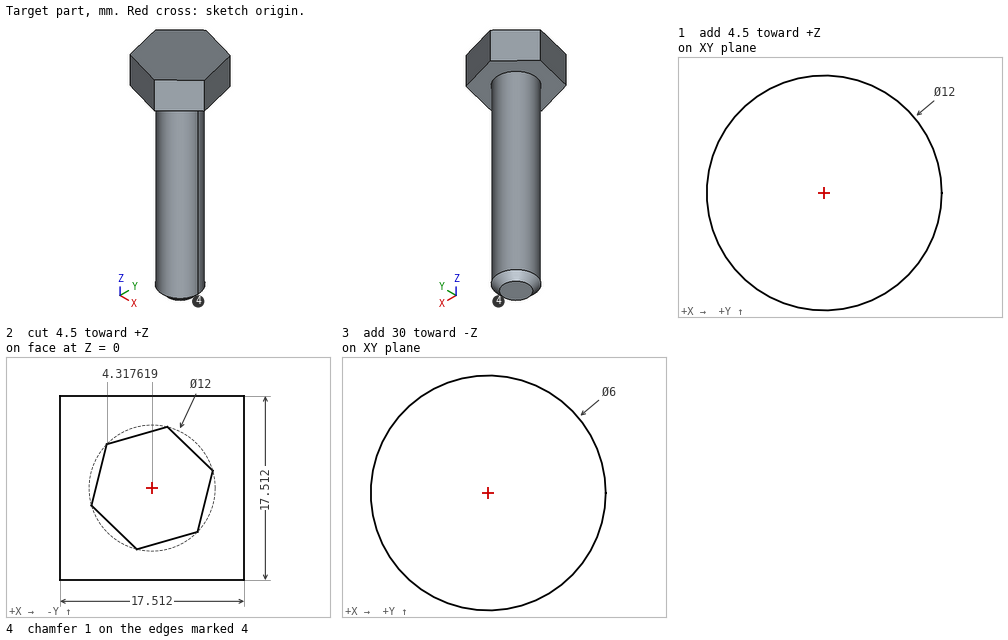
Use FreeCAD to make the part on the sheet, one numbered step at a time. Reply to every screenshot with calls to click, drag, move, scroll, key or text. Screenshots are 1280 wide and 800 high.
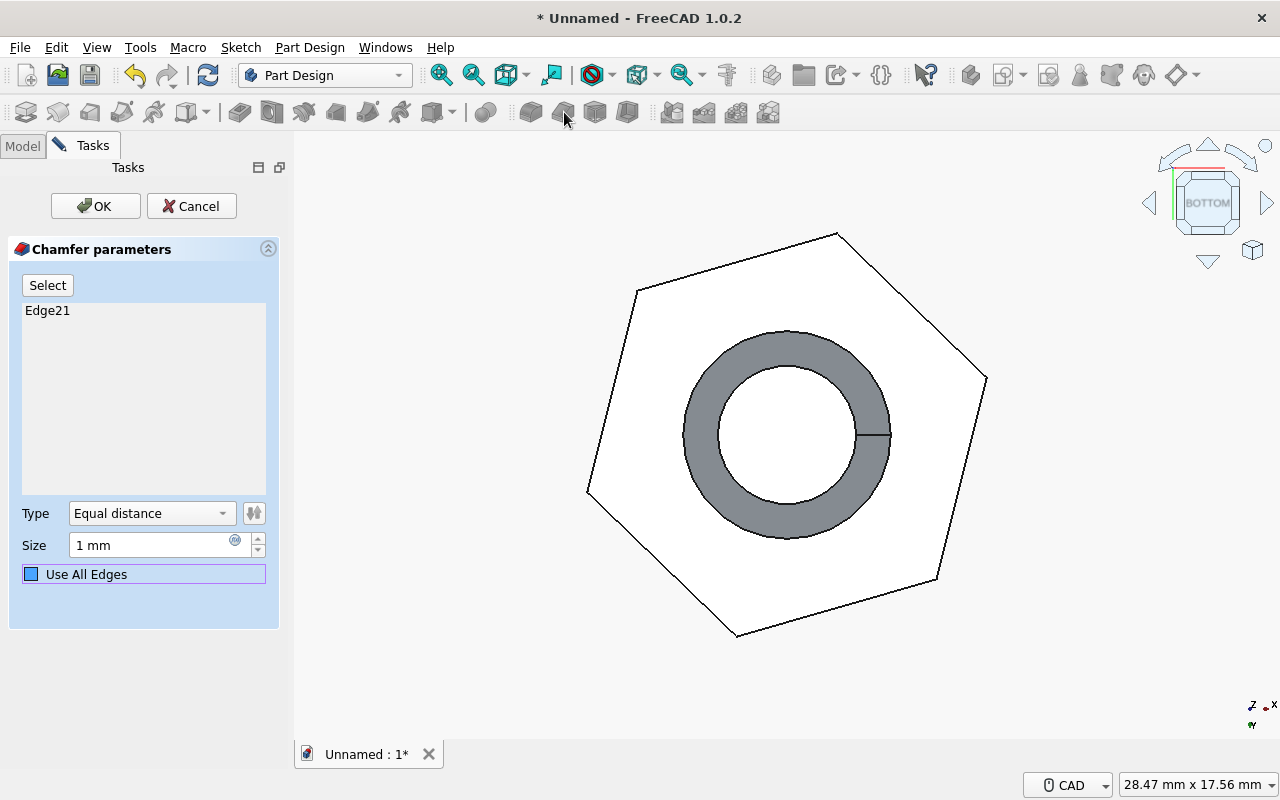
click(96, 206)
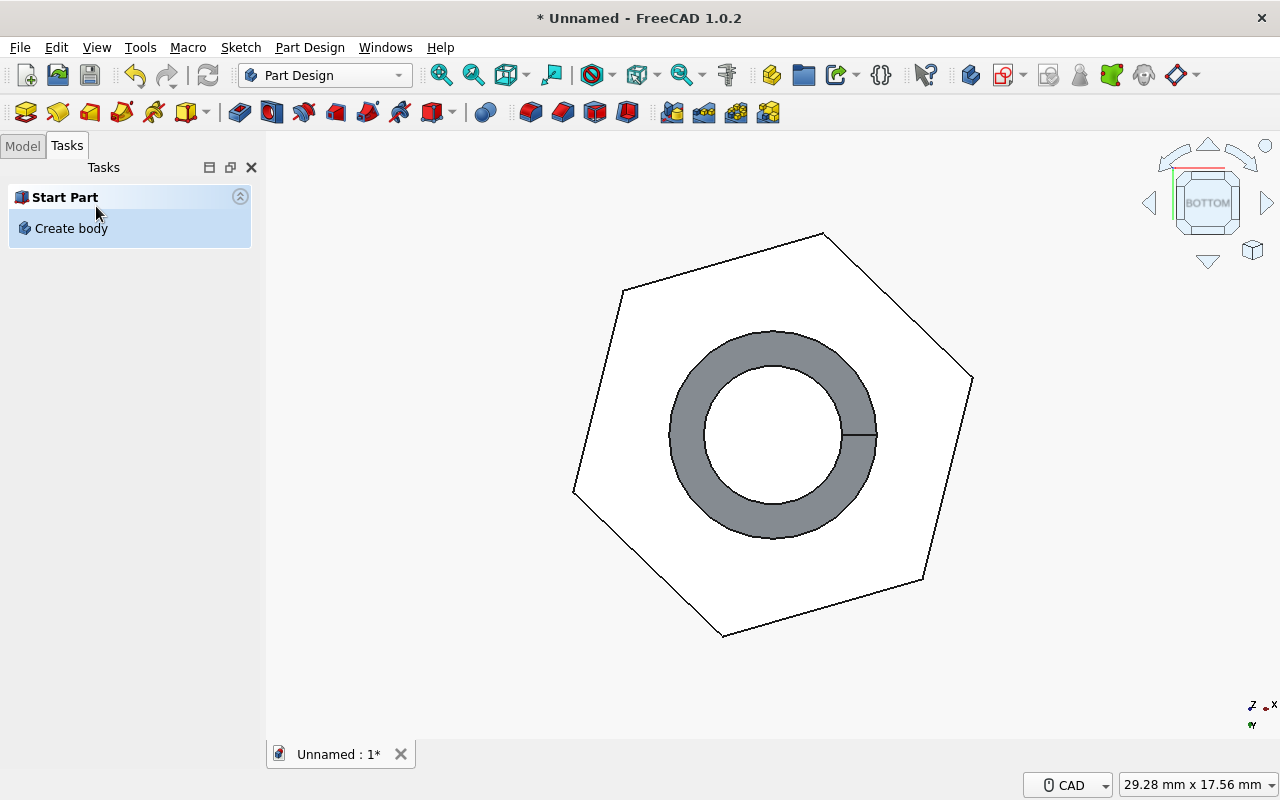
key(0)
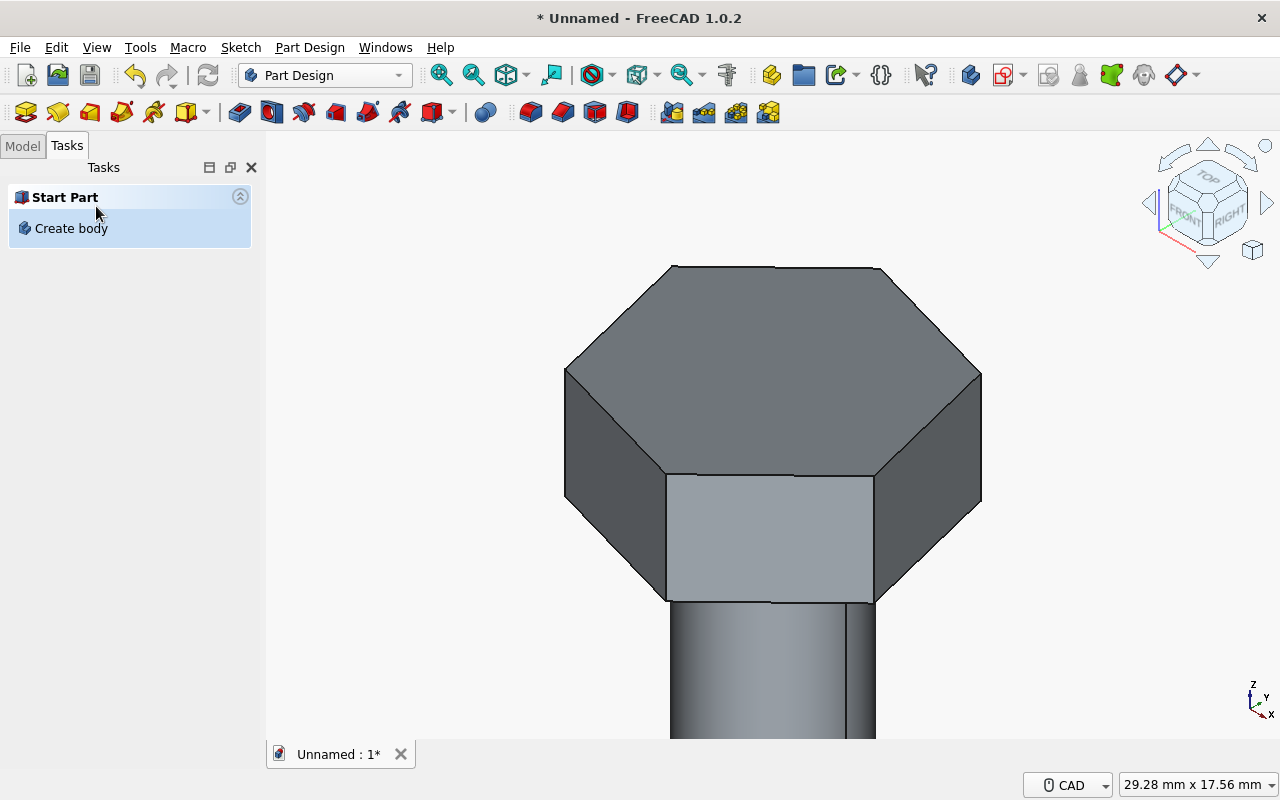
key(v)
key(f)